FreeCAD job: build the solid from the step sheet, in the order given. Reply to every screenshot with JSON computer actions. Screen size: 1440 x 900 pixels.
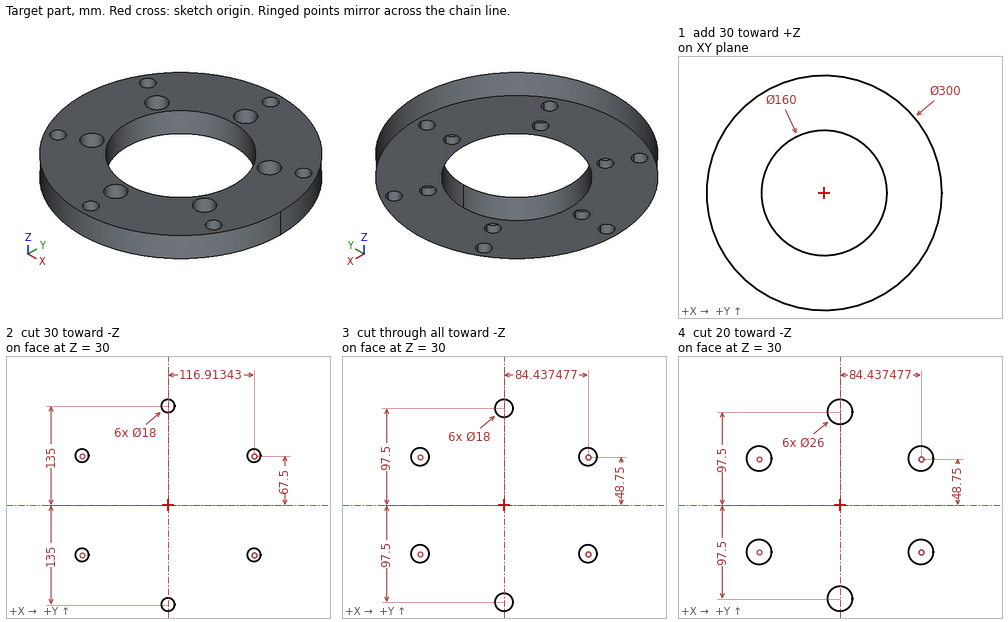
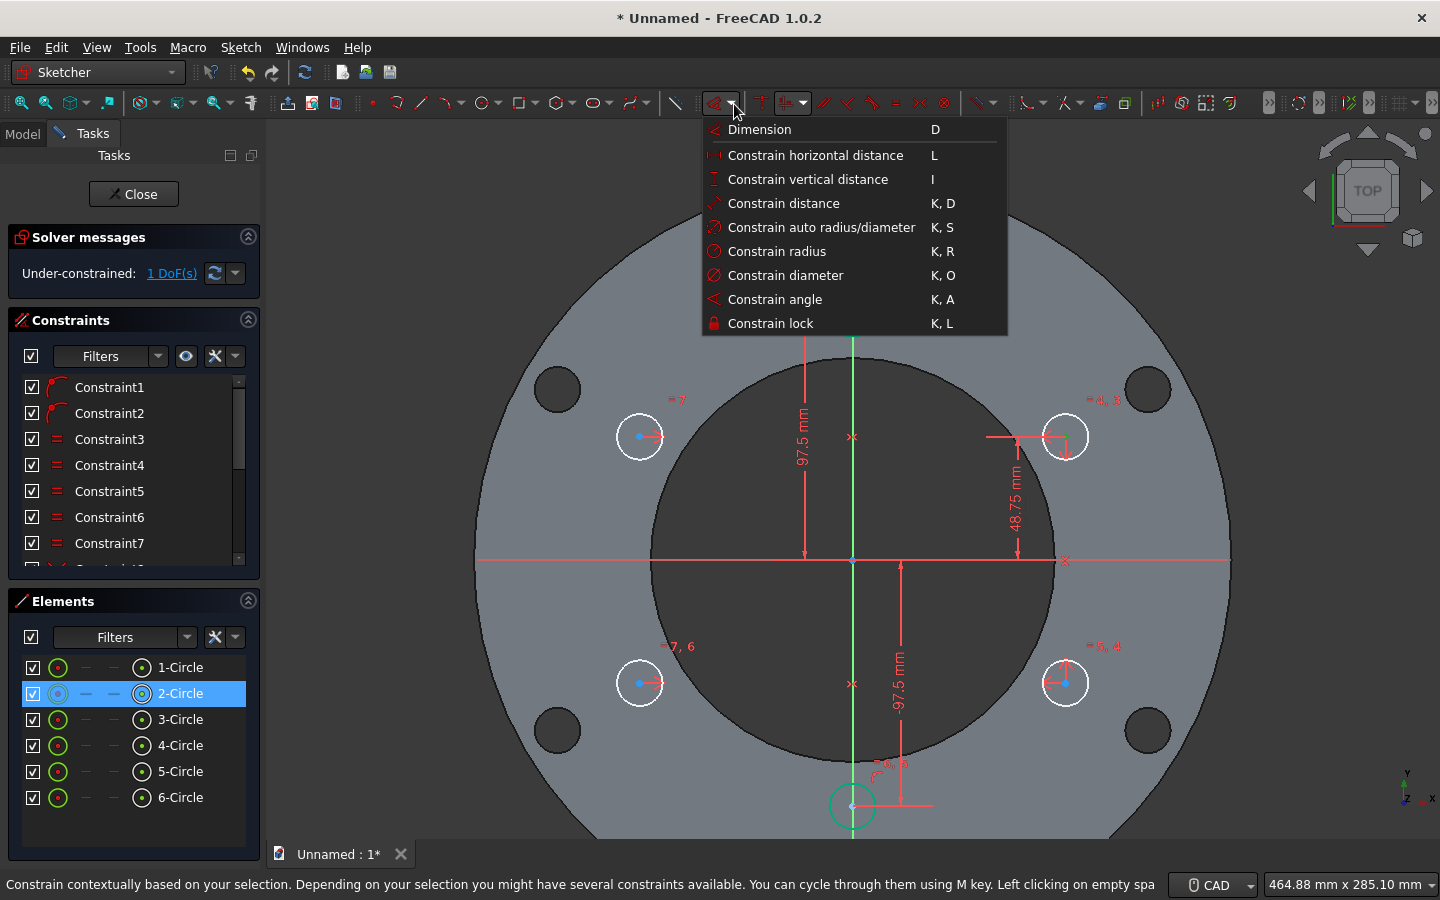
{"action": "left_click", "coordinate": [855, 155]}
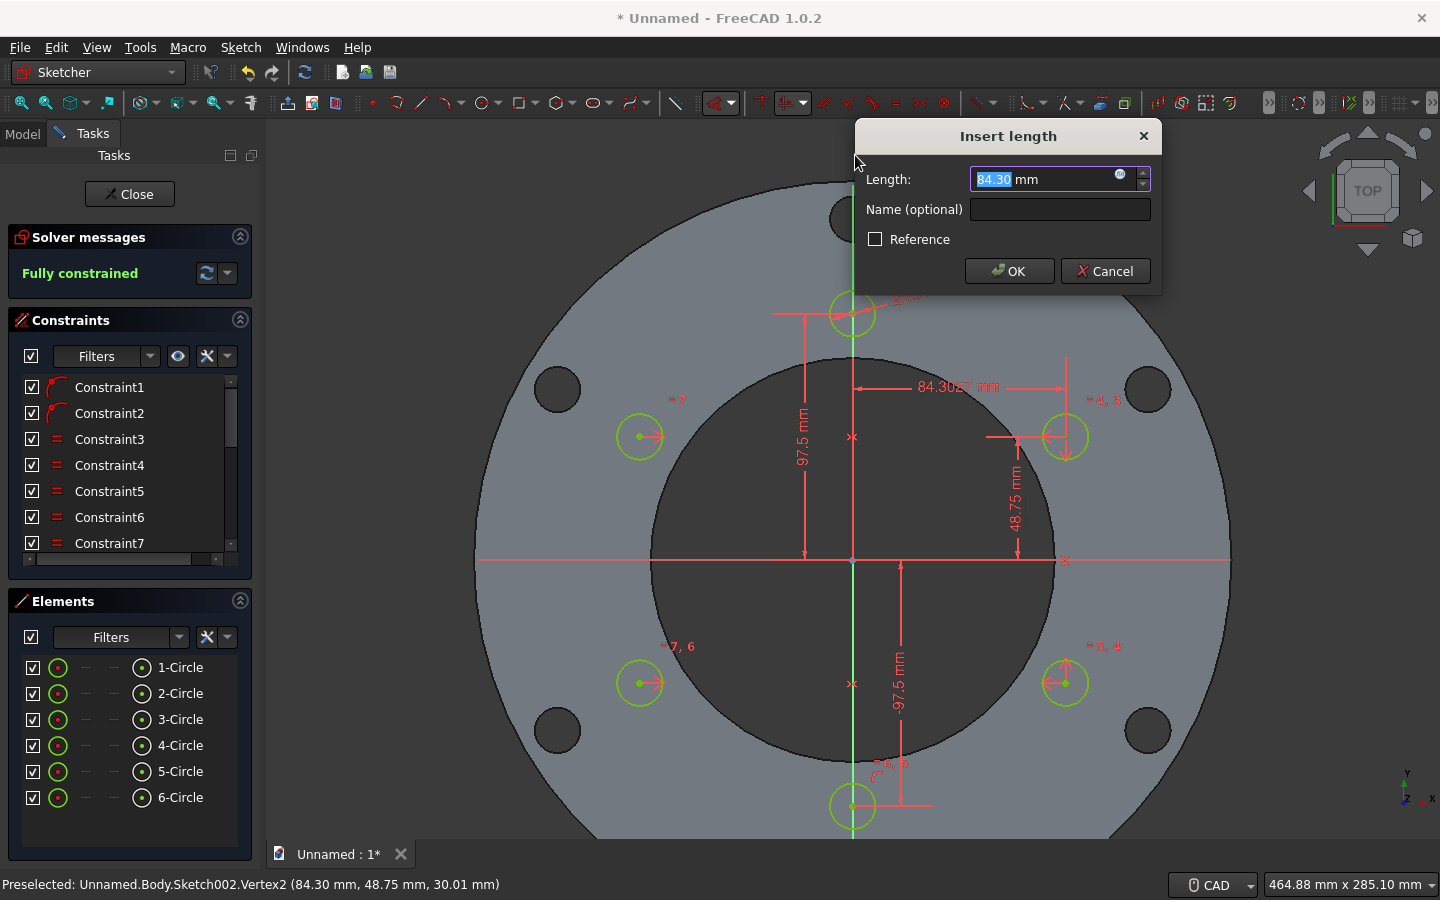
{"action": "type", "text": "84.437477"}
{"action": "key", "text": "Return"}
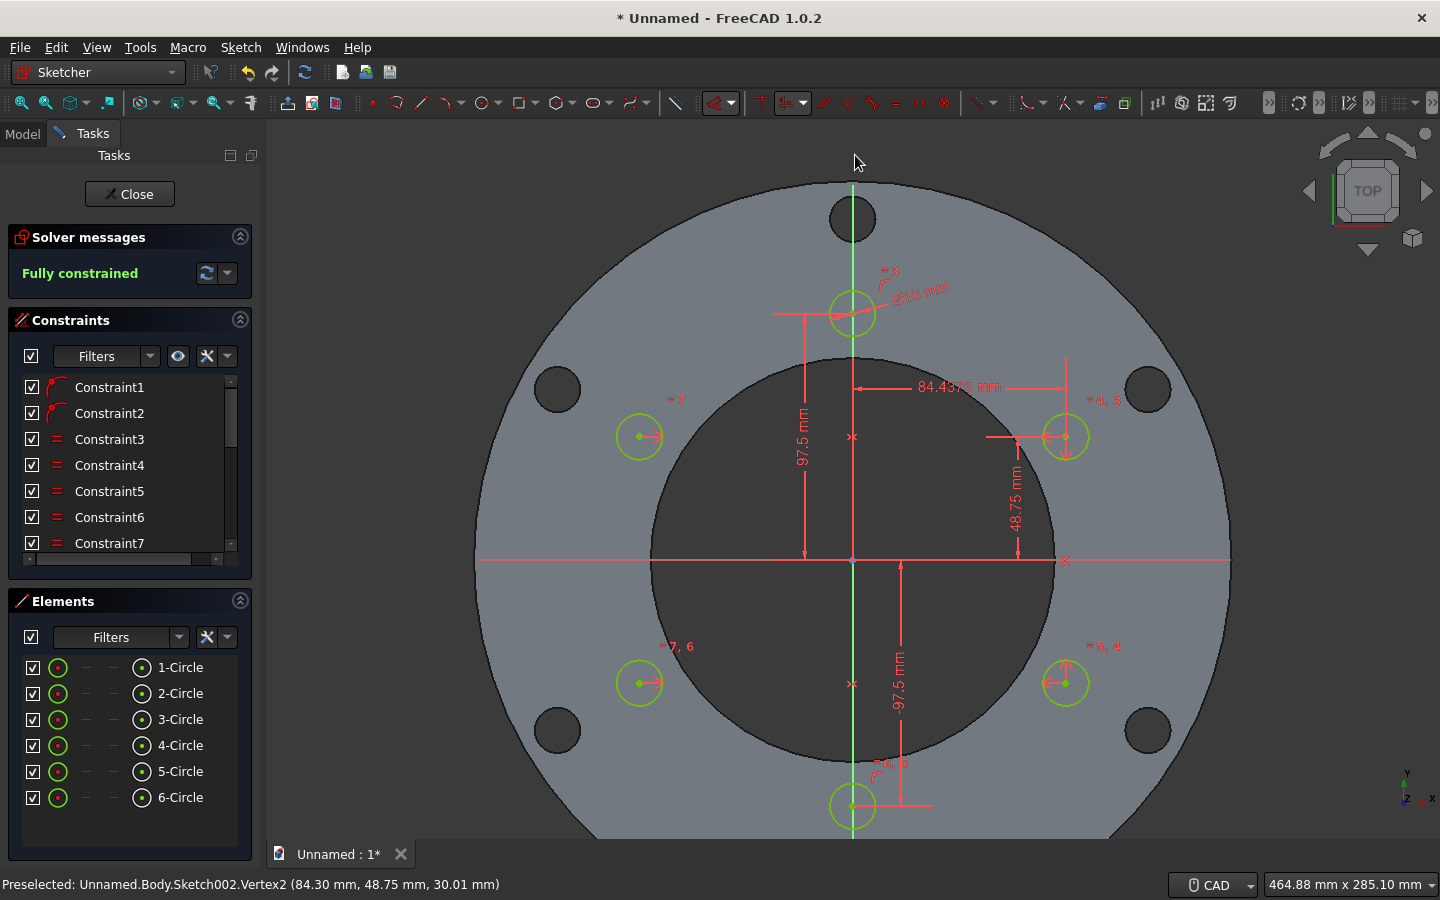
{"action": "left_click", "coordinate": [130, 194]}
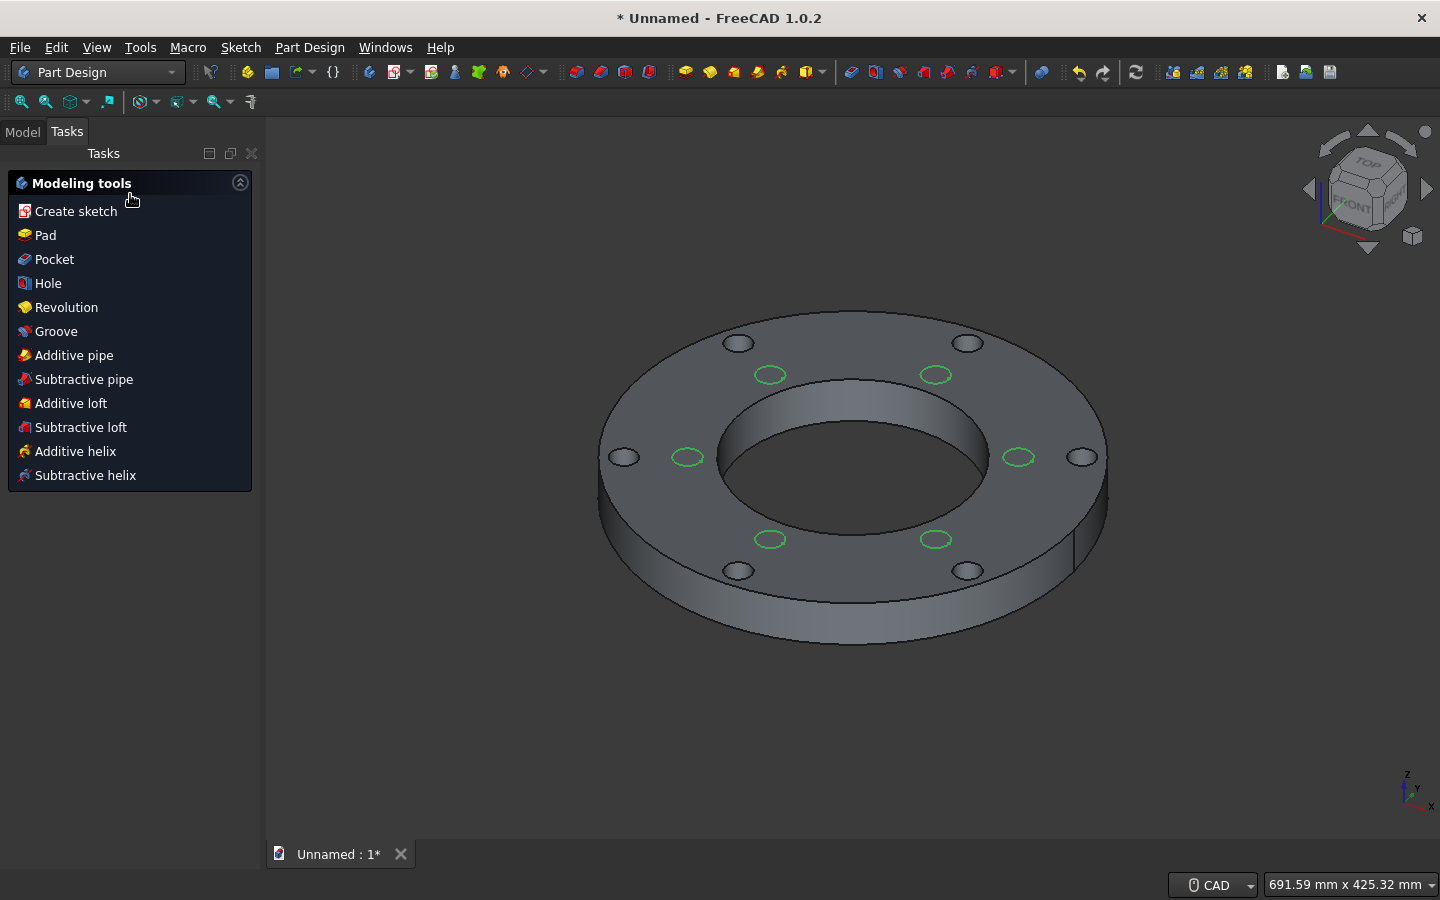
{"action": "left_click", "coordinate": [852, 72]}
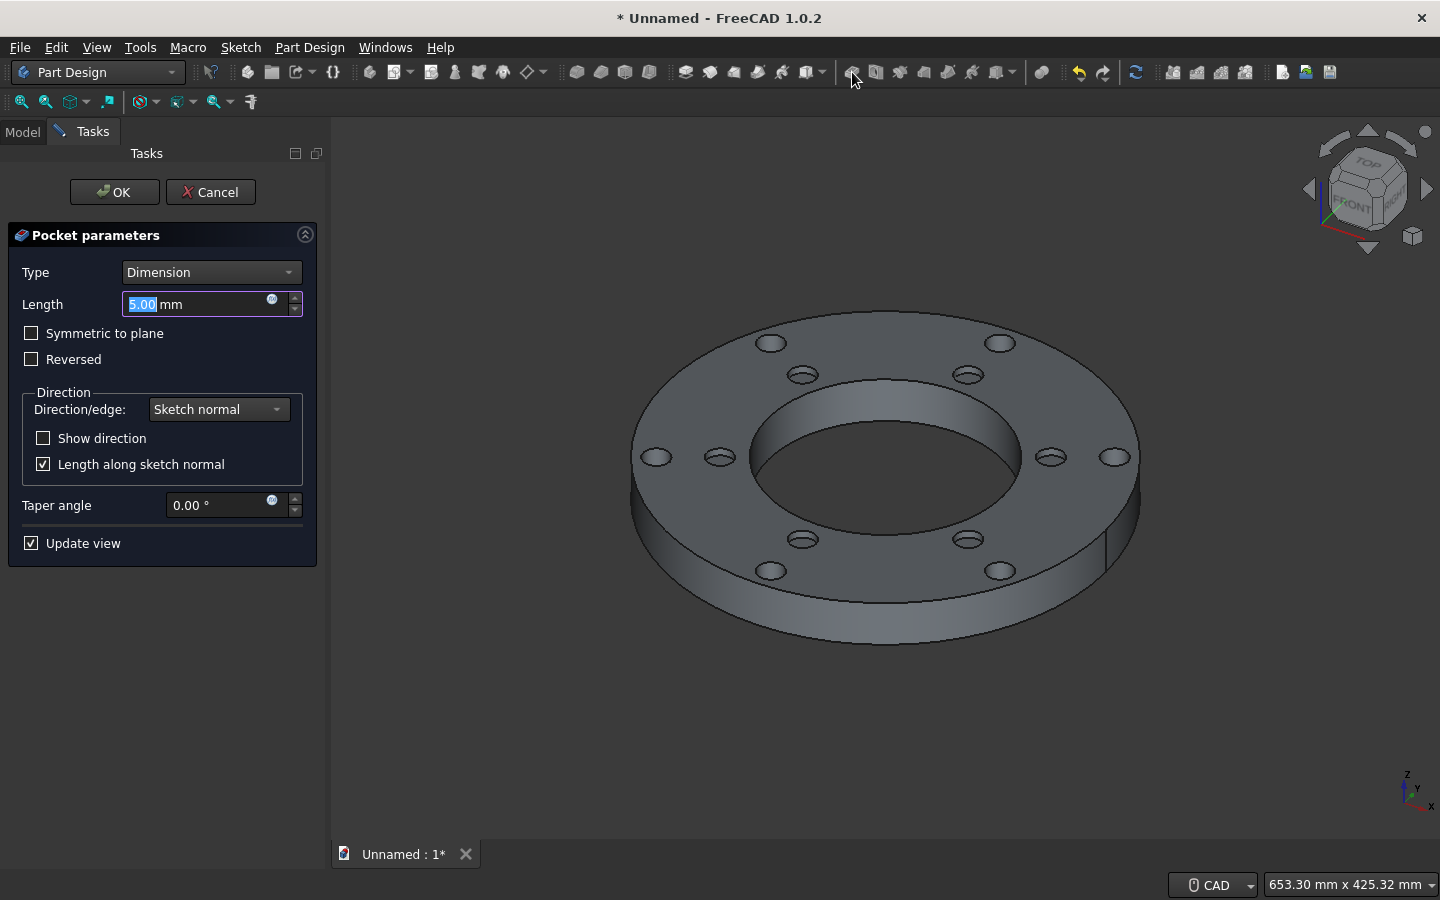
{"action": "left_click", "coordinate": [212, 272]}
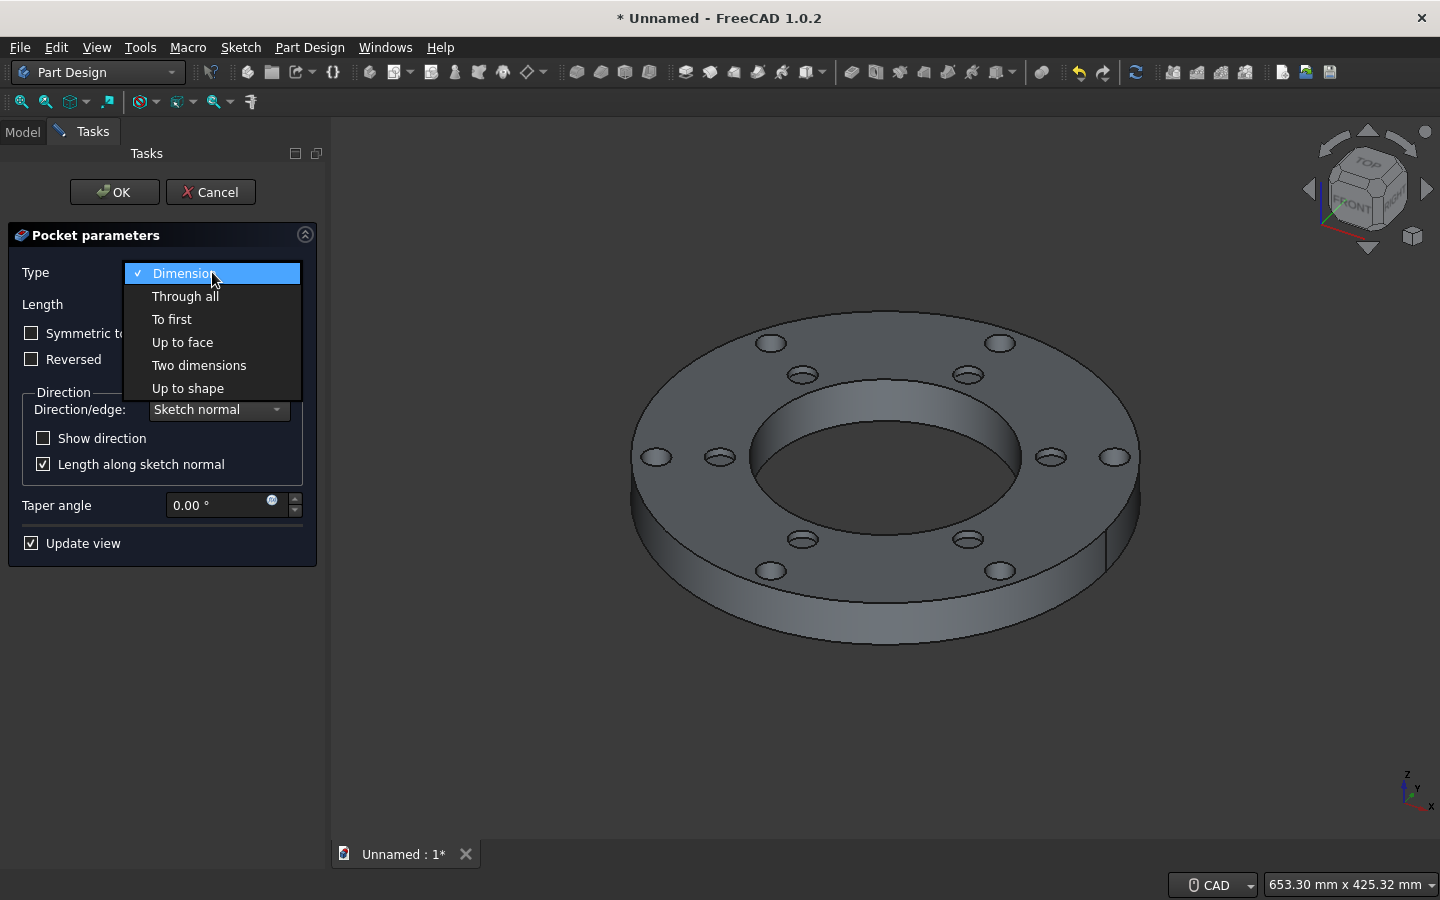
{"action": "left_click", "coordinate": [212, 296]}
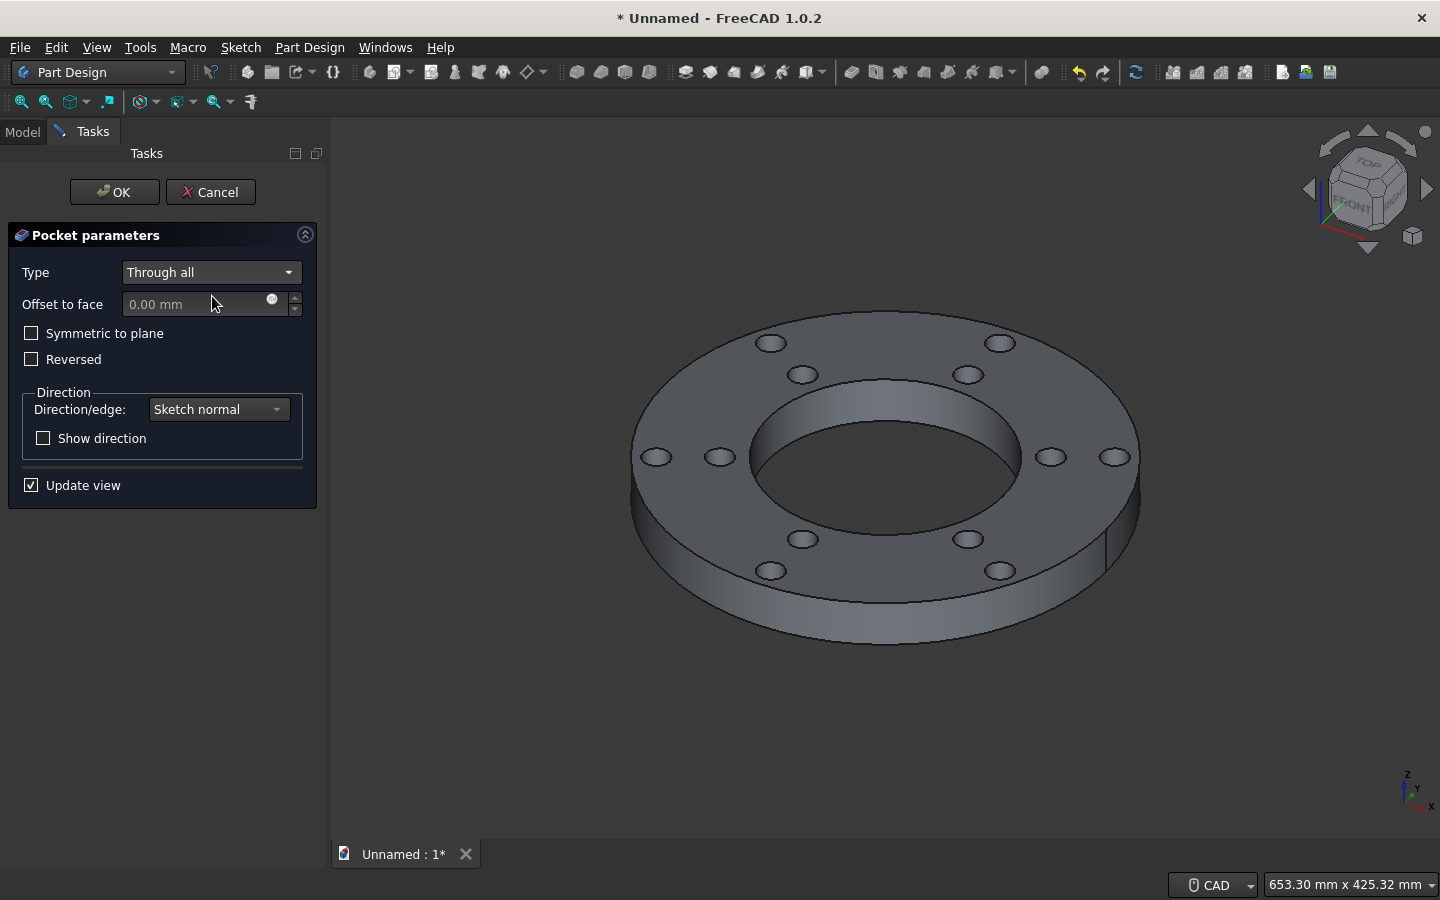
{"action": "left_click", "coordinate": [115, 192]}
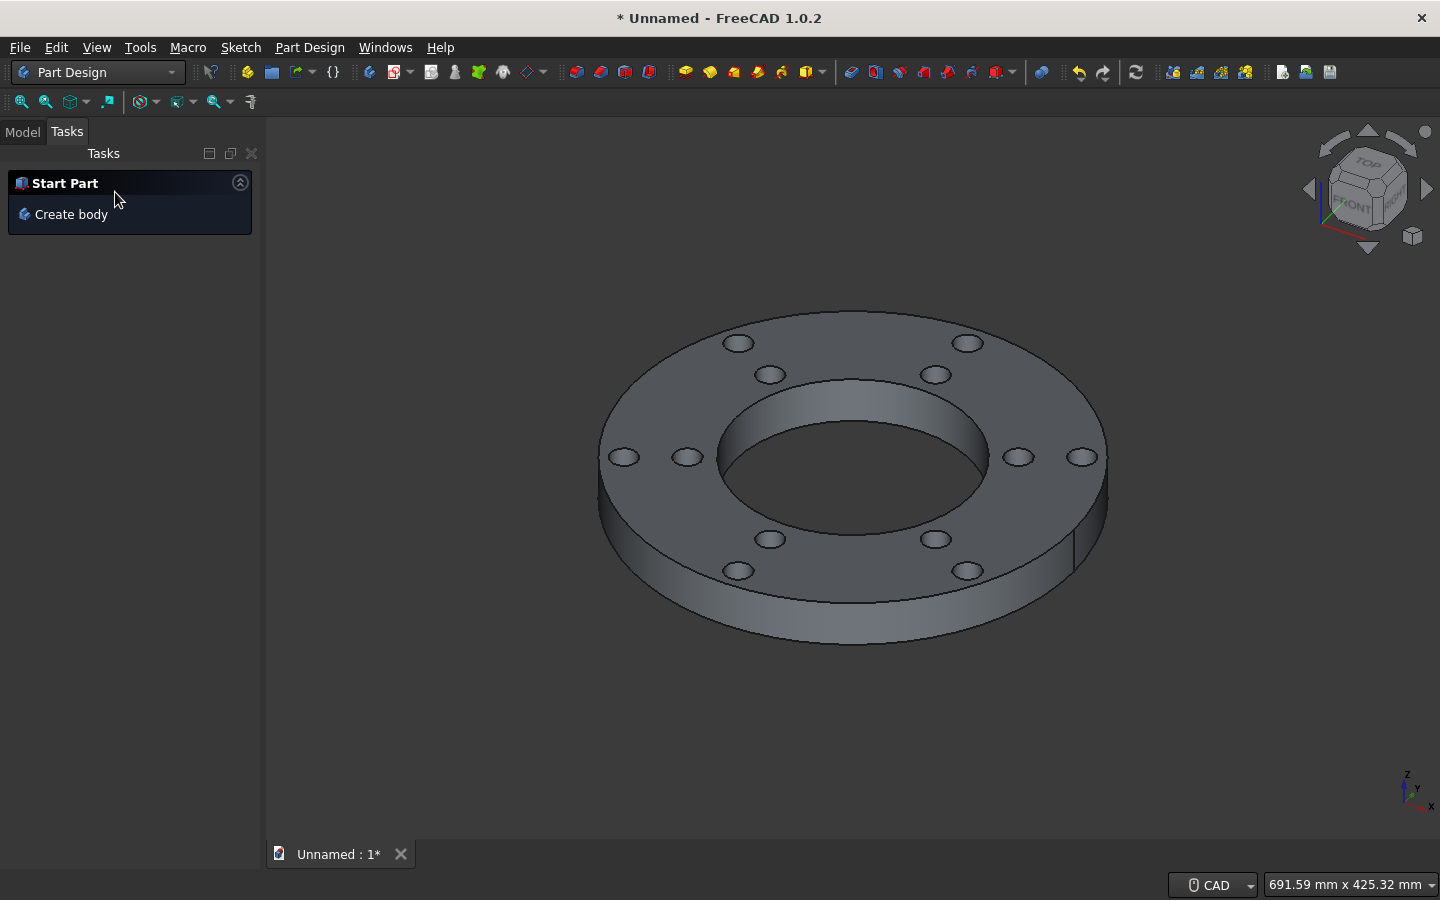
{"action": "left_click", "coordinate": [1052, 426]}